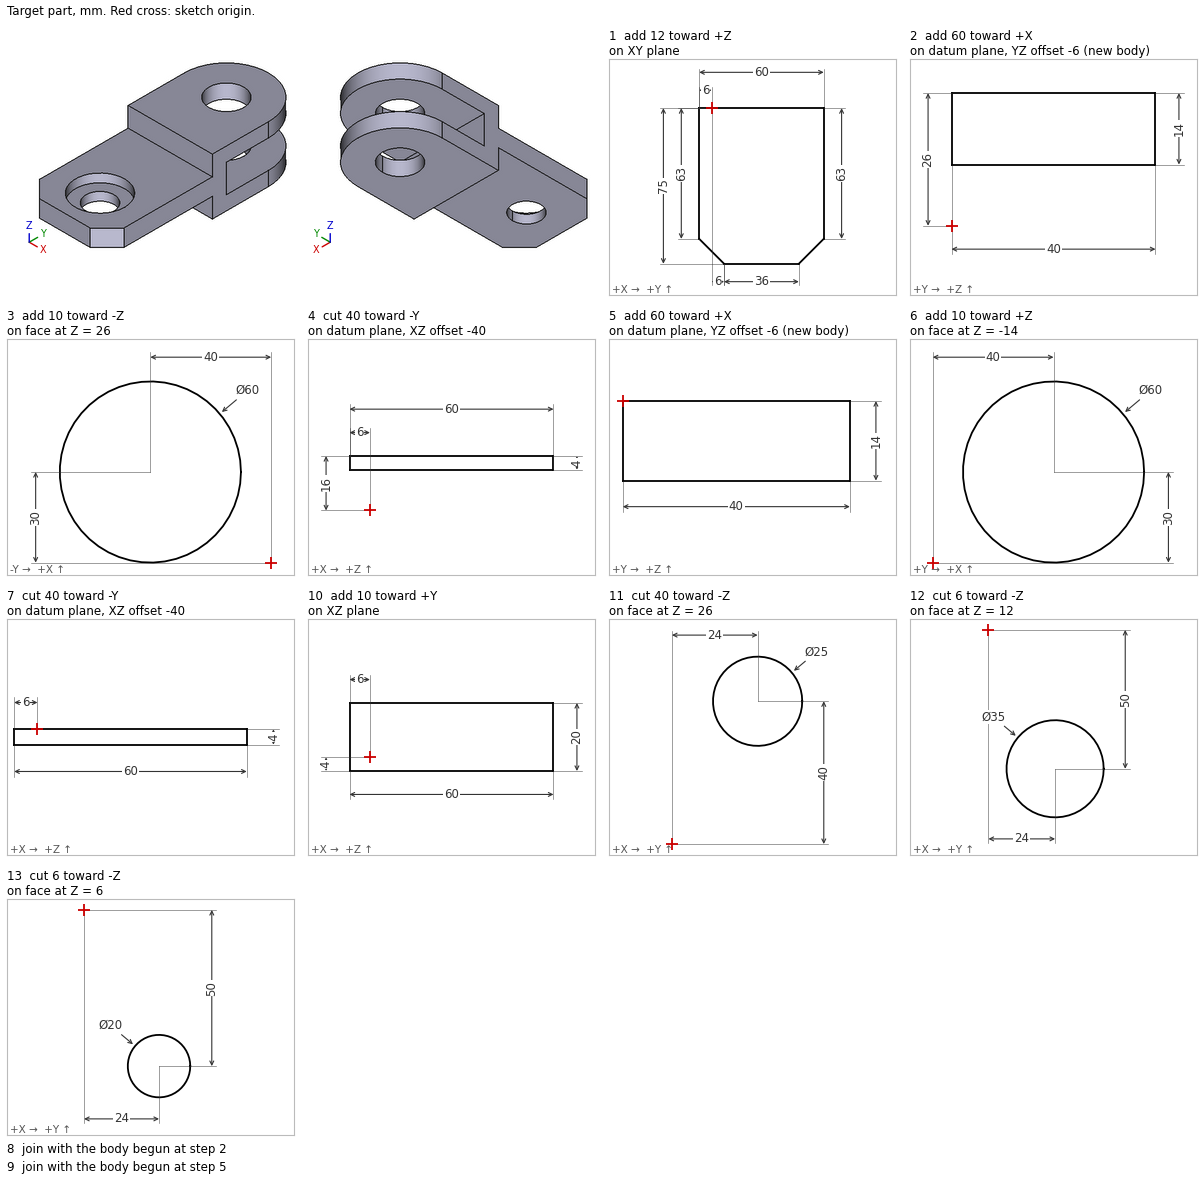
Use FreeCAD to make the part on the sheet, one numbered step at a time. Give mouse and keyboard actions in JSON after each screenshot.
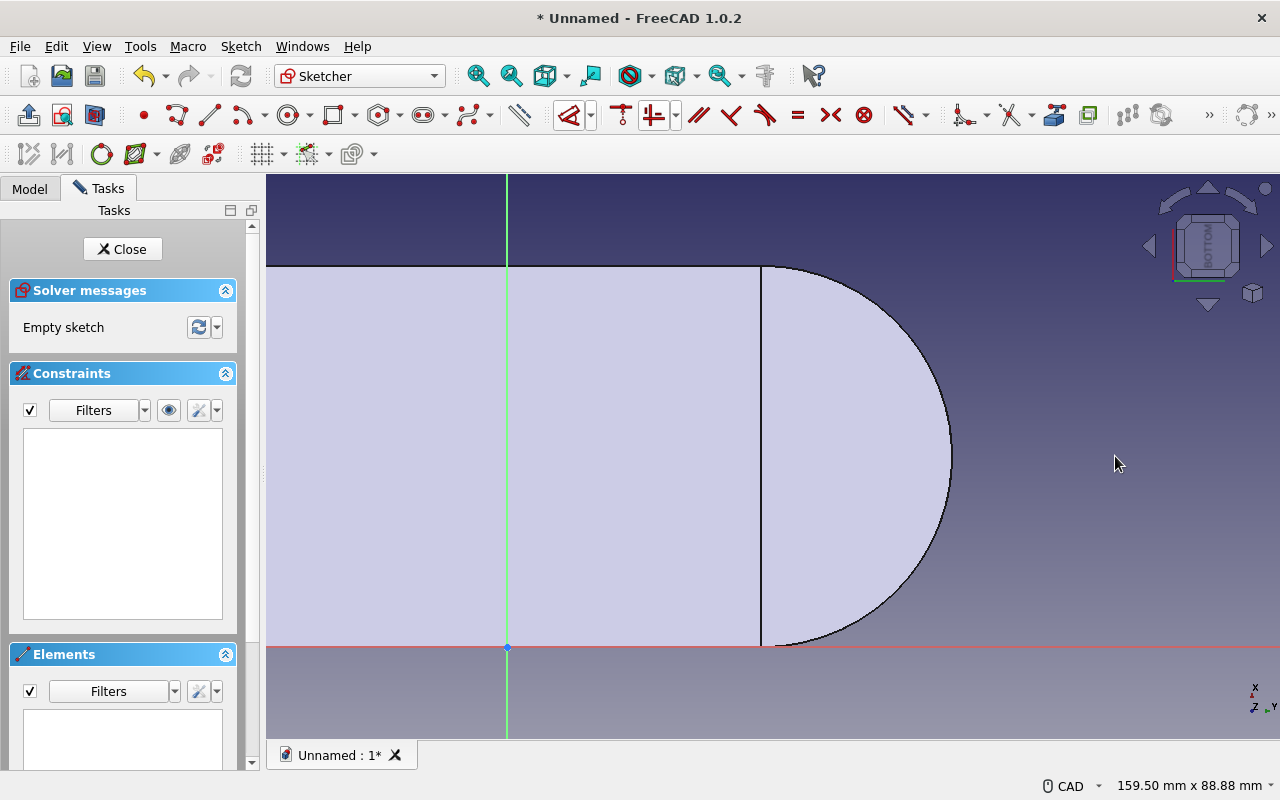
{"action": "left_click", "coordinate": [288, 116]}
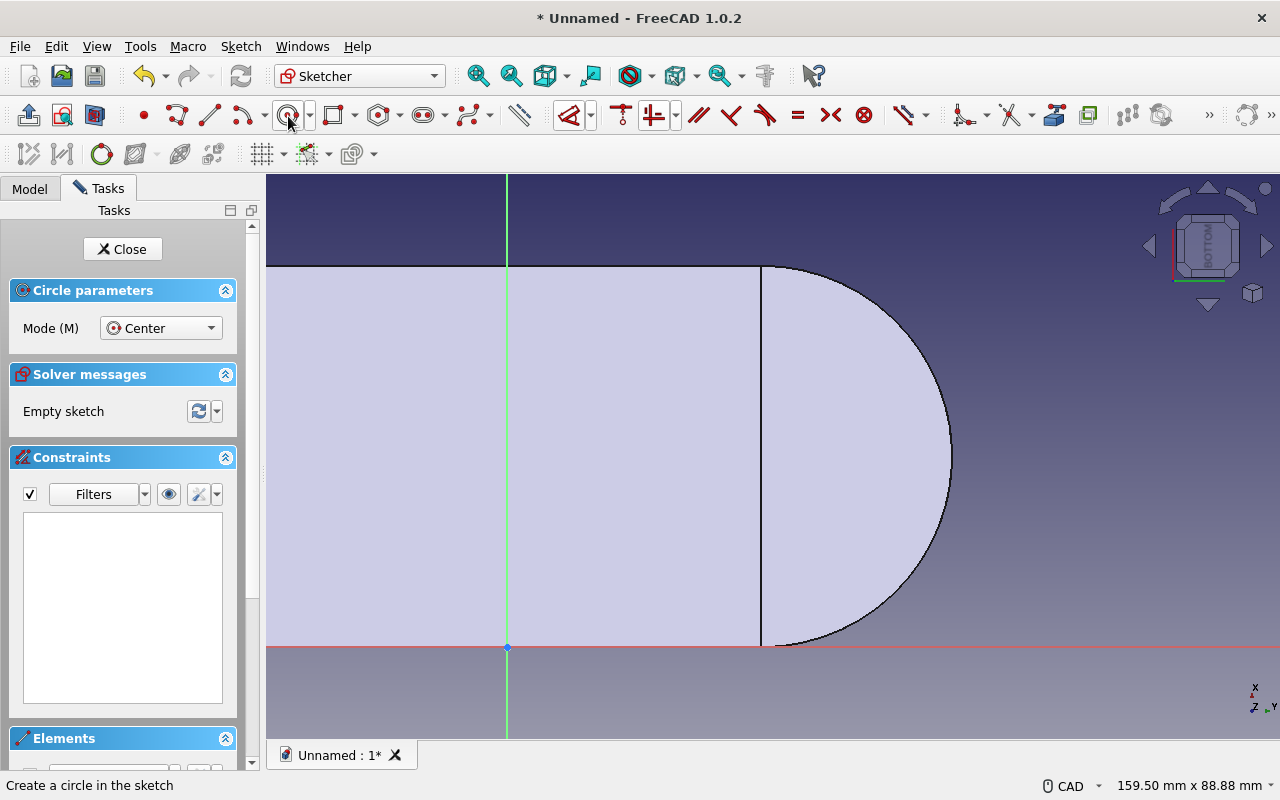
{"action": "left_click", "coordinate": [761, 456]}
{"action": "mouse_move", "coordinate": [896, 322]}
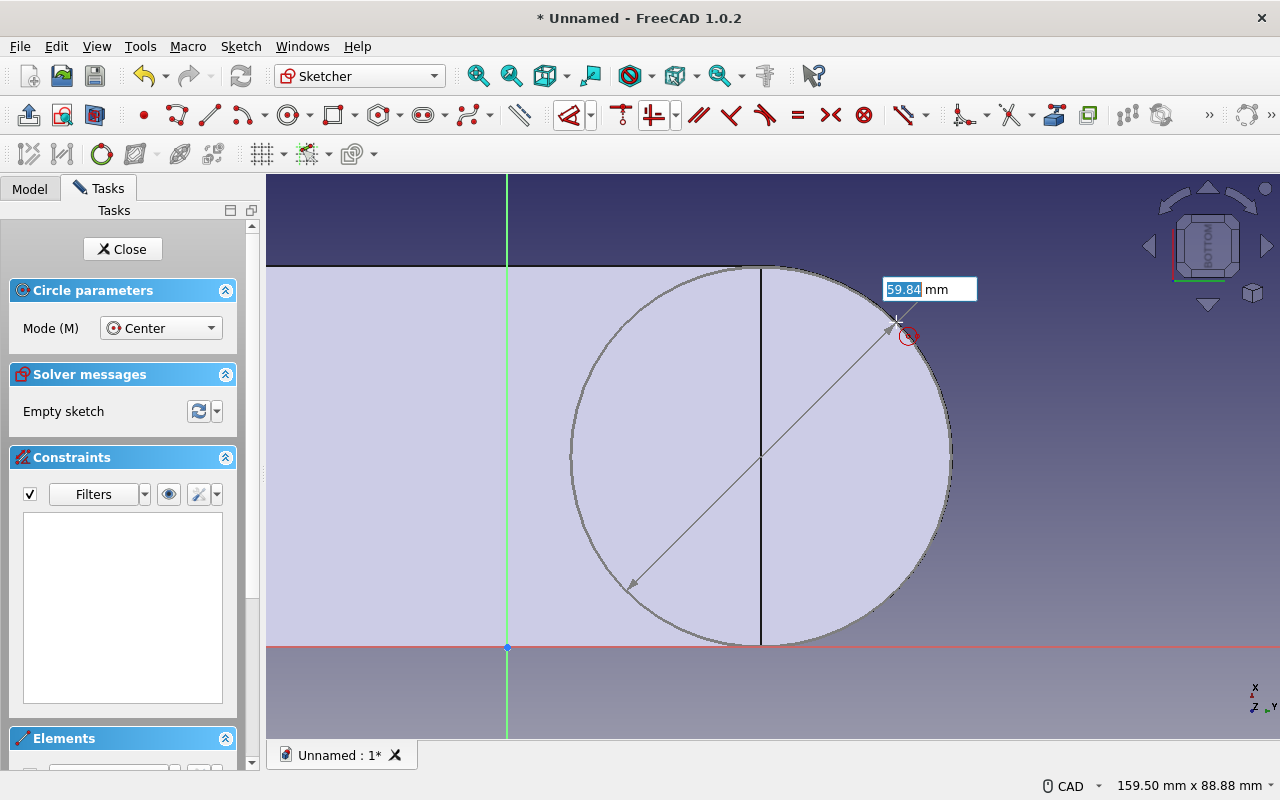
{"action": "type", "text": "60"}
{"action": "key", "text": "Return"}
{"action": "key", "text": "Escape"}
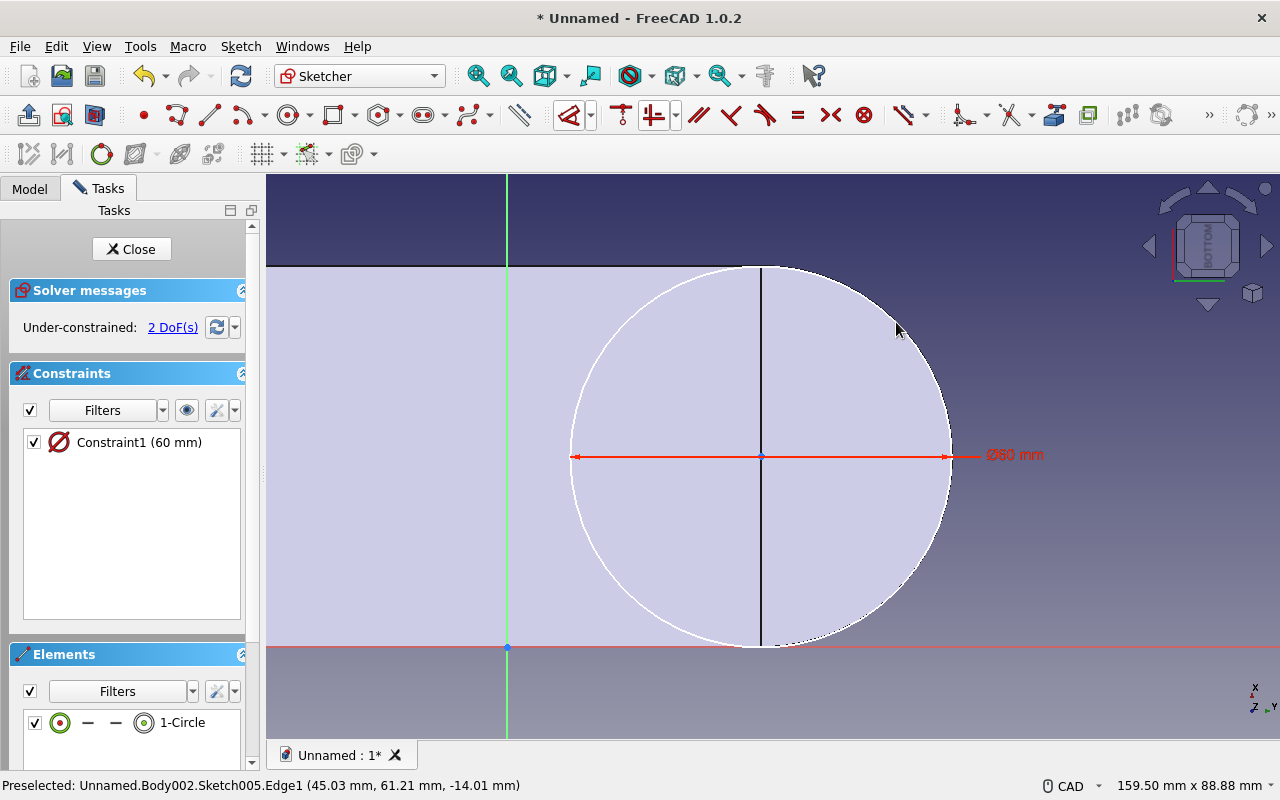
{"action": "left_click", "coordinate": [761, 457]}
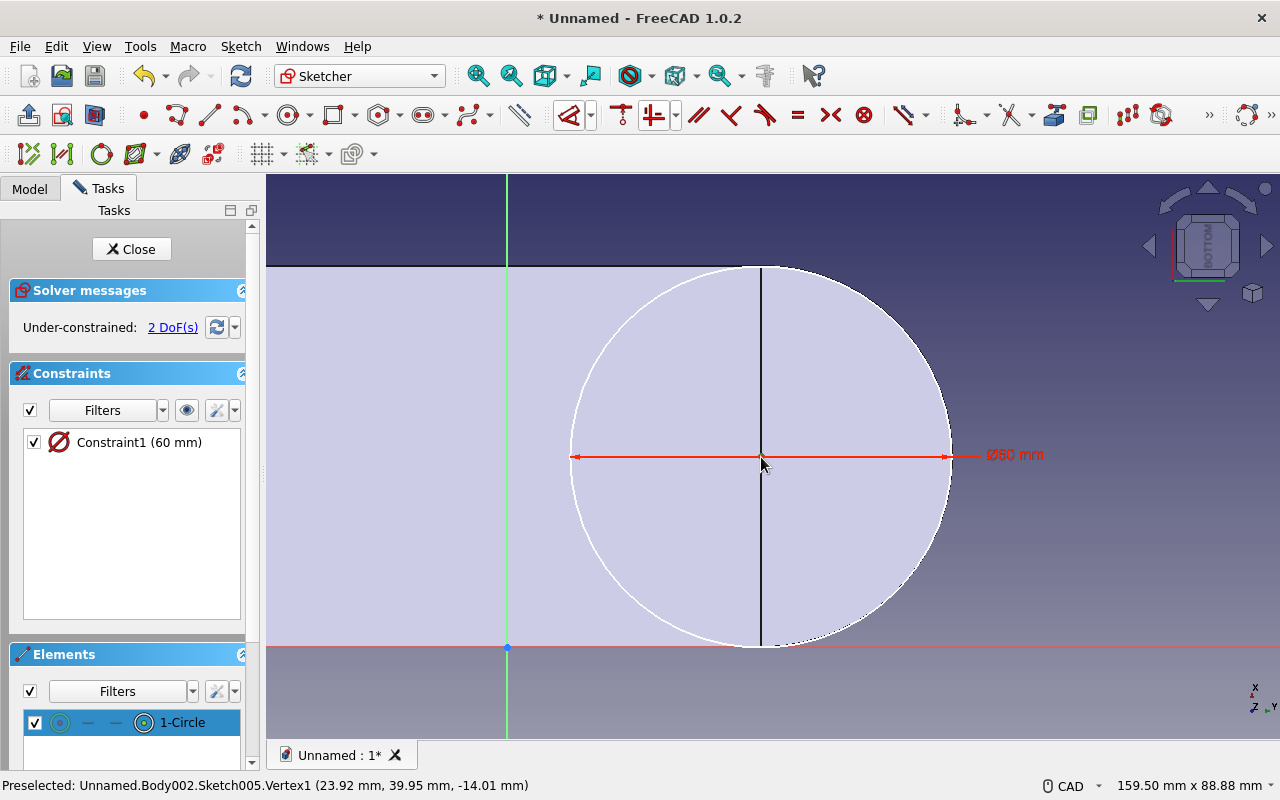
{"action": "key", "text": "l"}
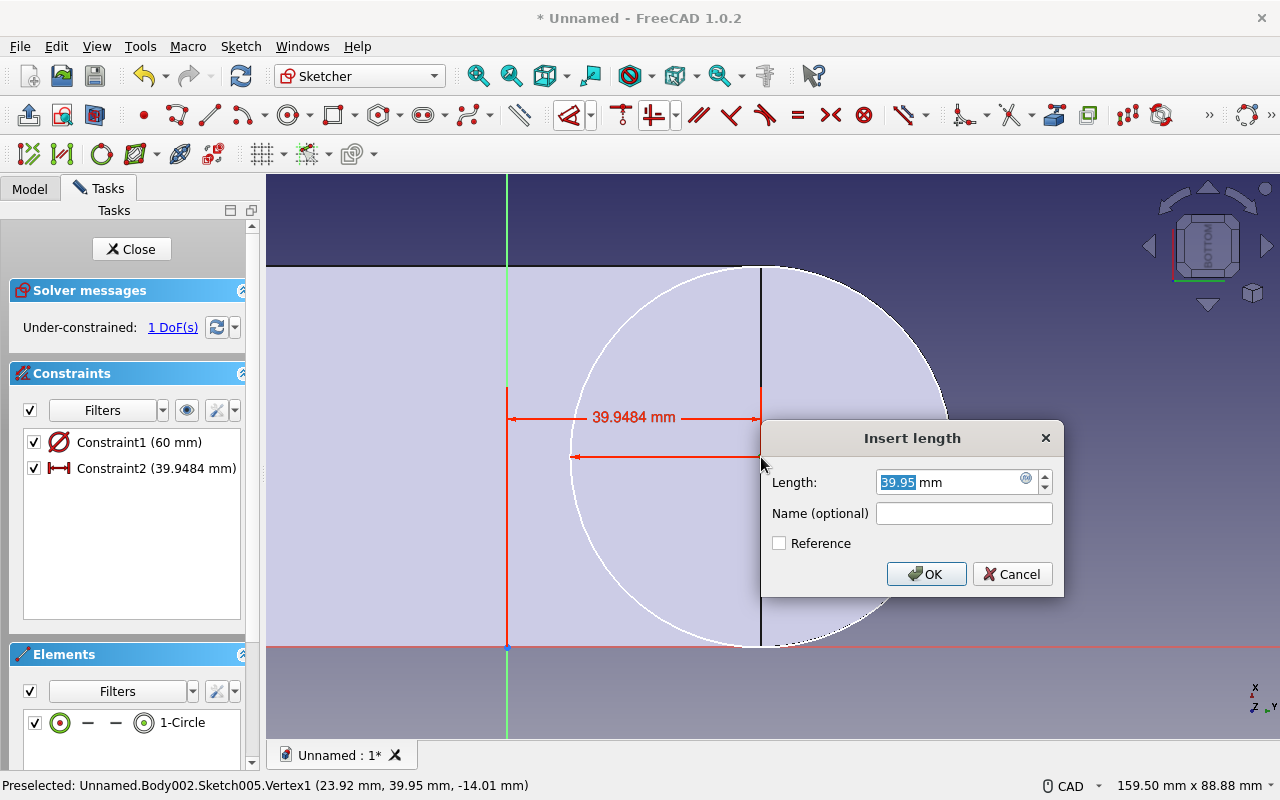
{"action": "type", "text": "40"}
{"action": "key", "text": "Return"}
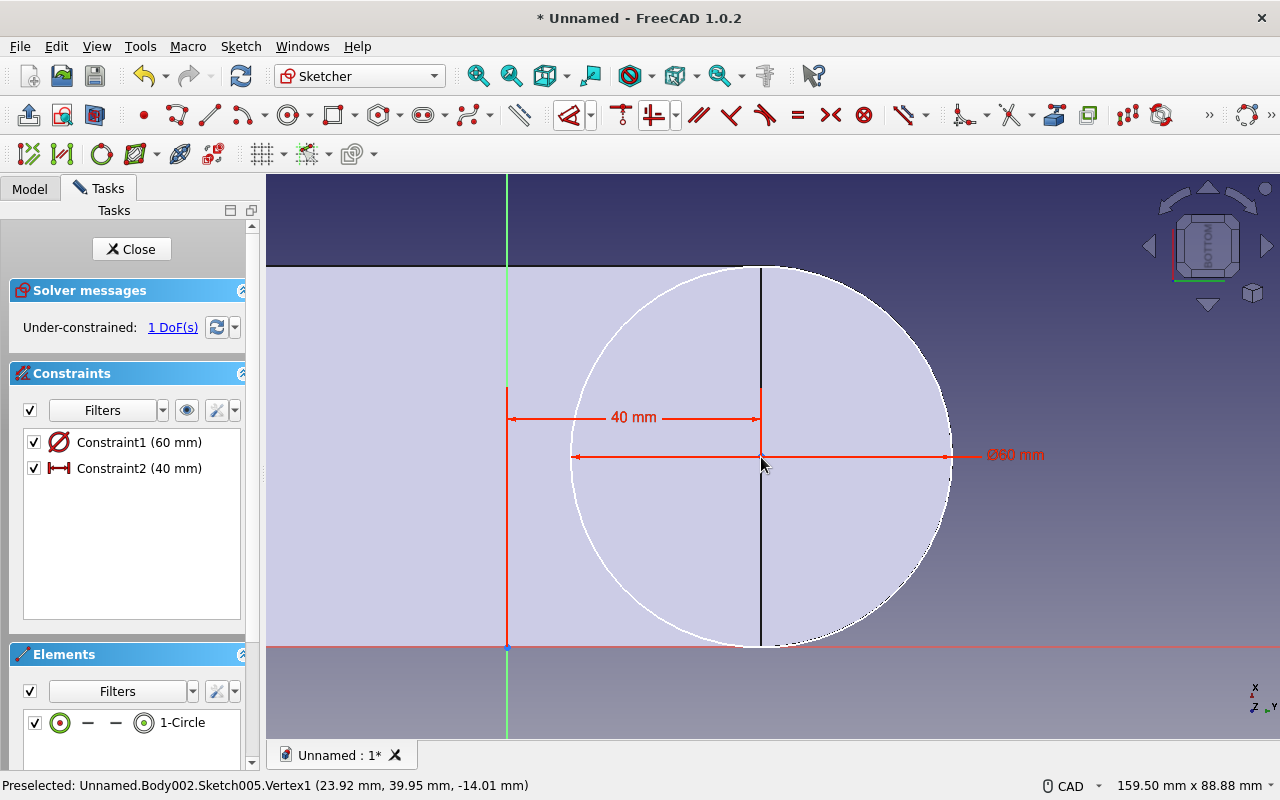
{"action": "left_click", "coordinate": [761, 457]}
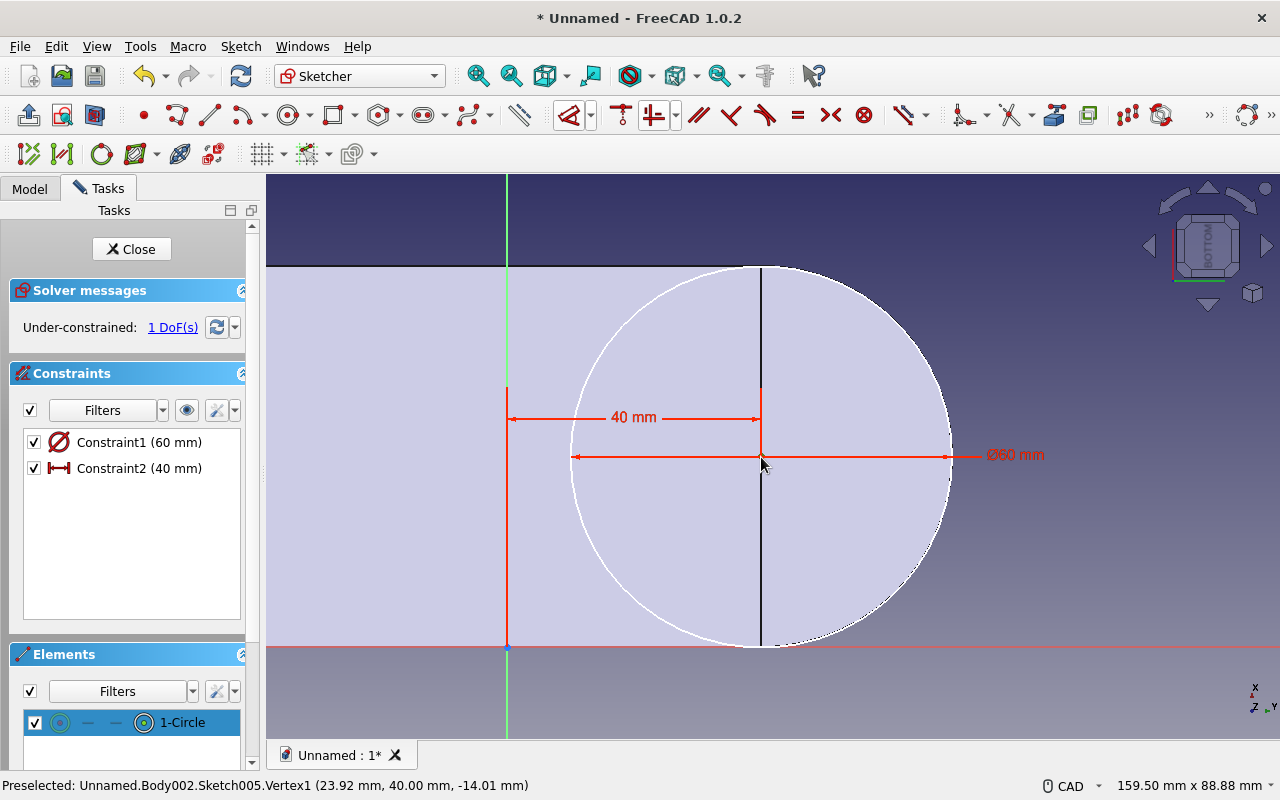
{"action": "key", "text": "i"}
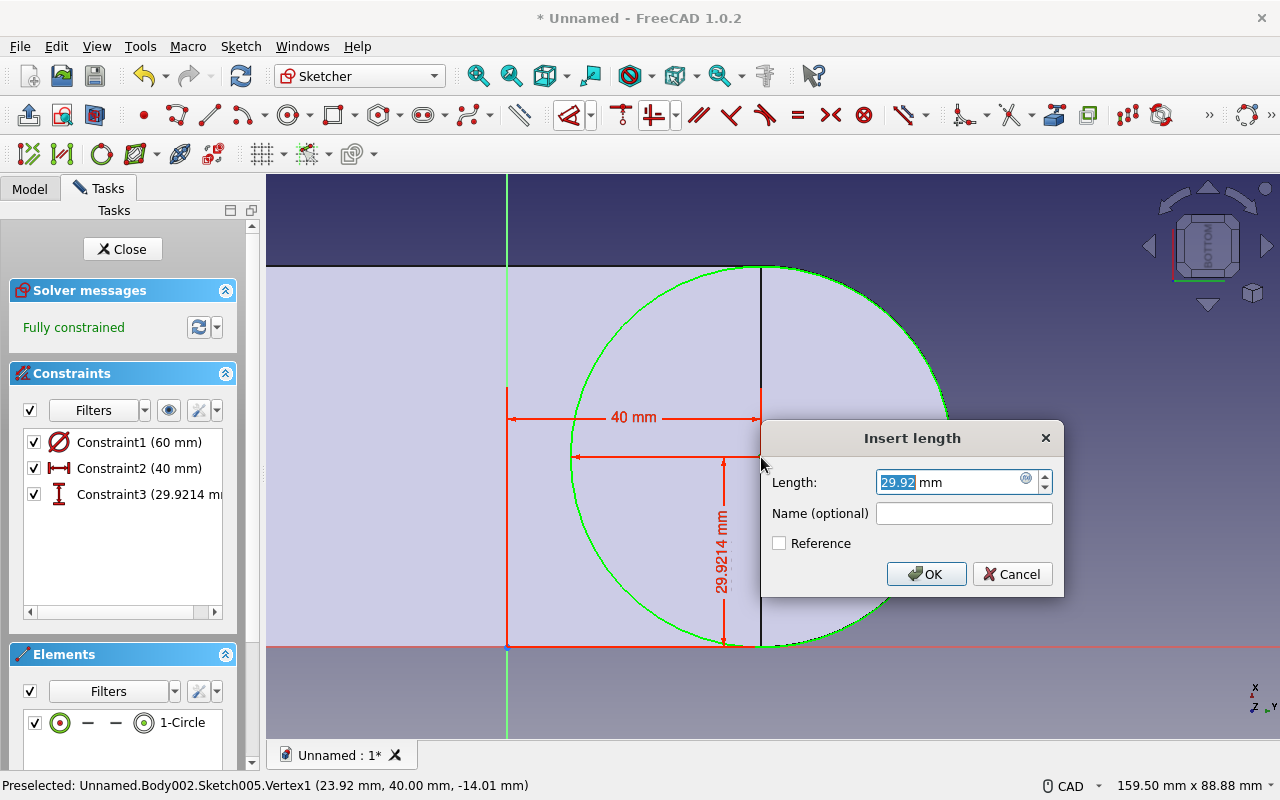
{"action": "type", "text": "30"}
{"action": "key", "text": "Return"}